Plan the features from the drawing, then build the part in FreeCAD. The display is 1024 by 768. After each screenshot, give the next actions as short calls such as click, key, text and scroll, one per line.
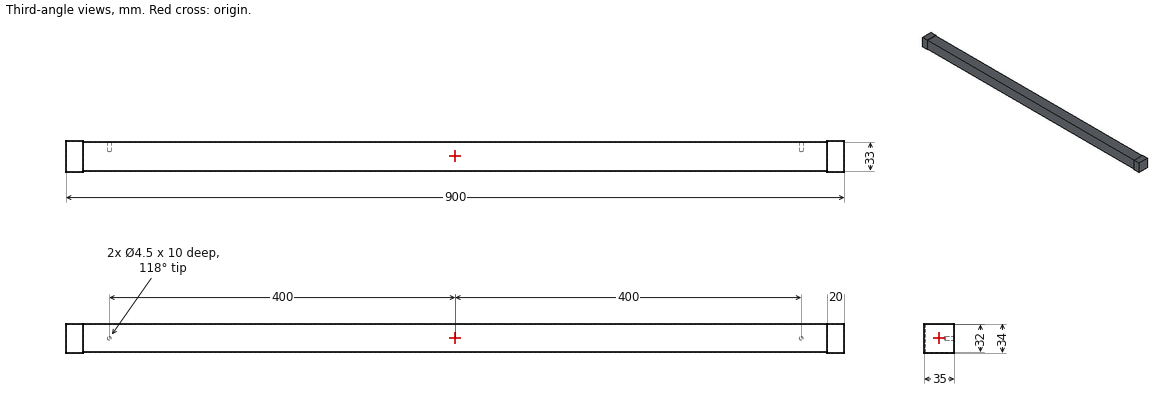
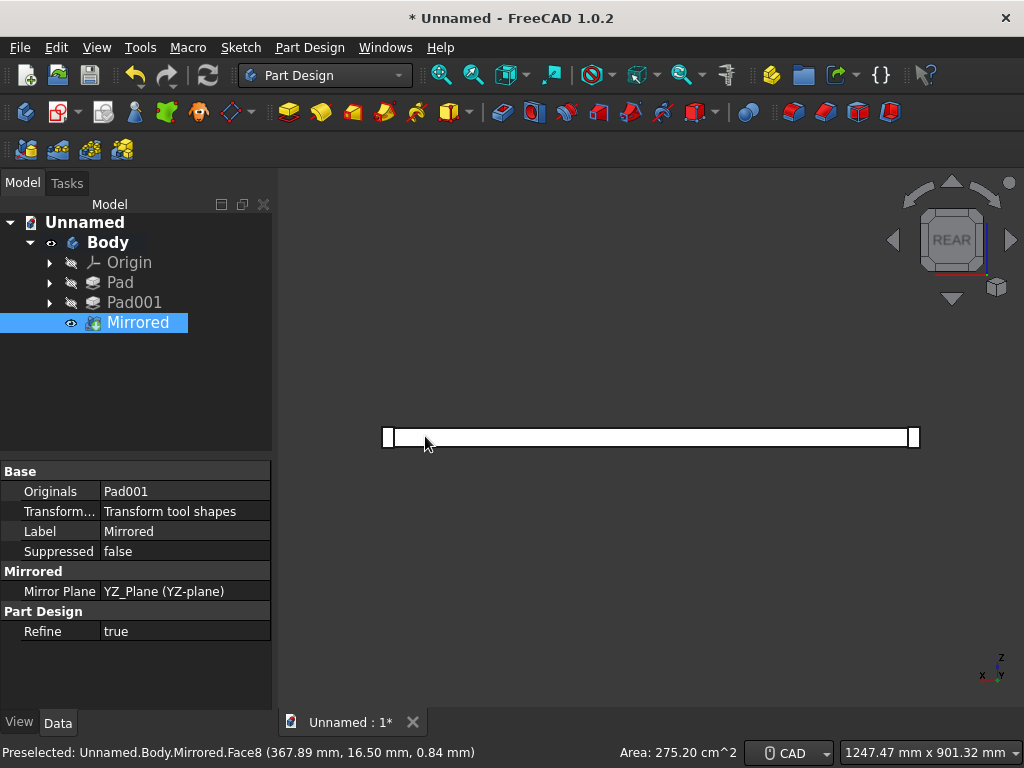
click(58, 112)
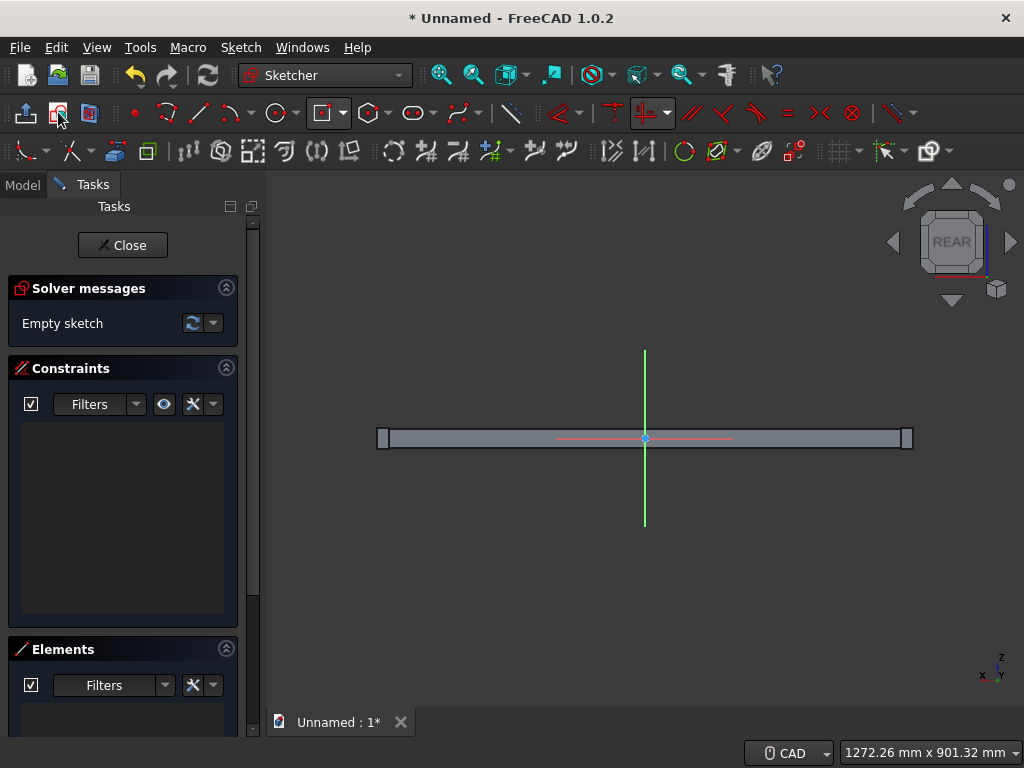
scroll(294, 439, down, 1)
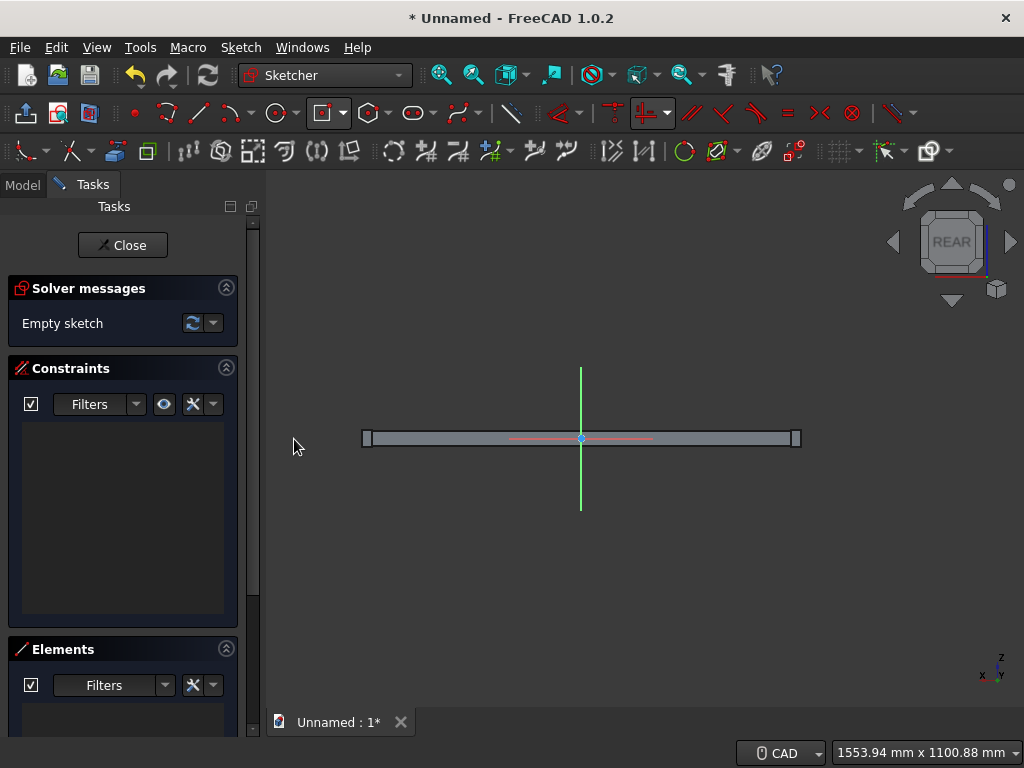
click(276, 114)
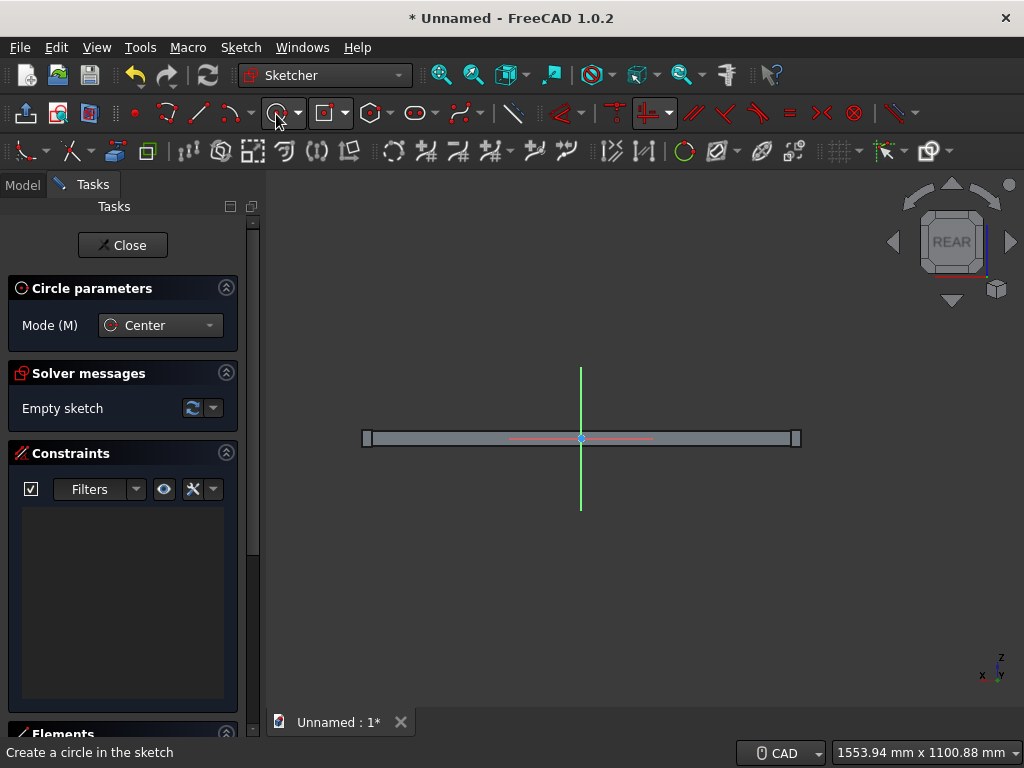
scroll(776, 439, up, 16)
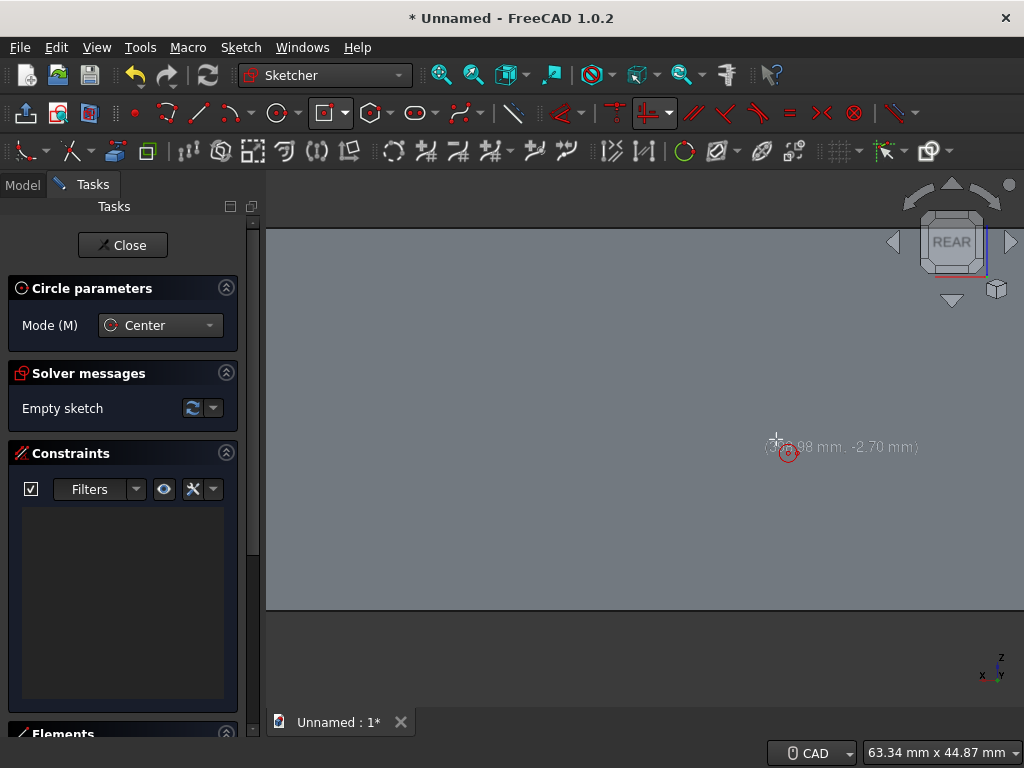
scroll(817, 440, down, 15)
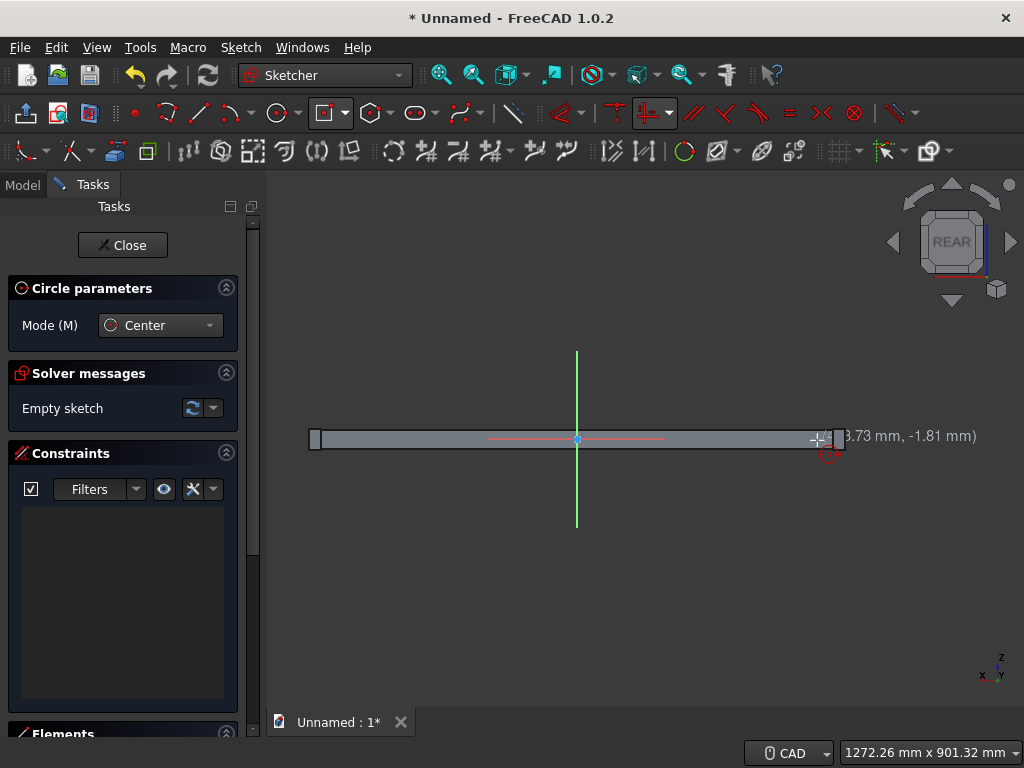
click(815, 439)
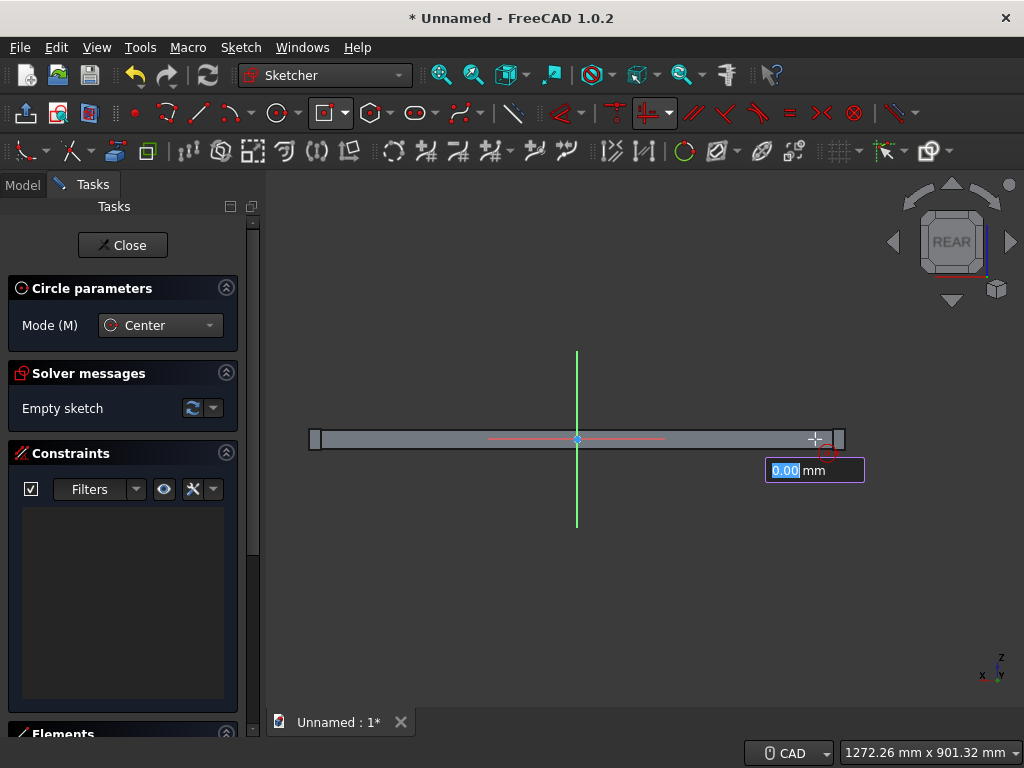
scroll(815, 441, up, 13)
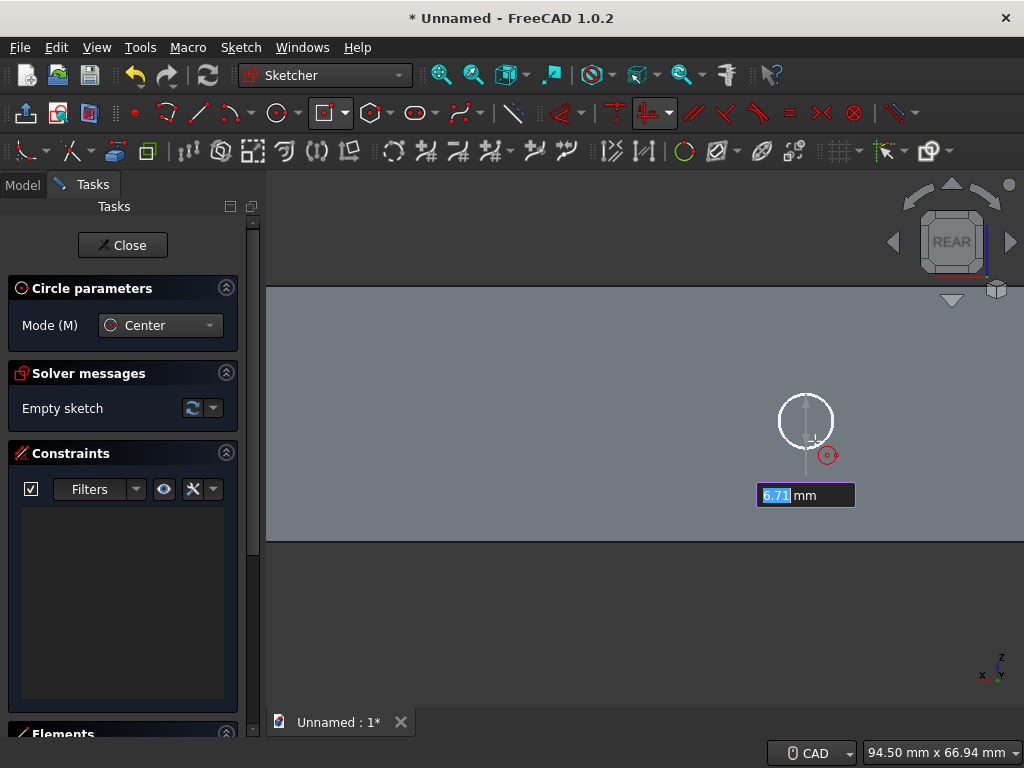
click(806, 431)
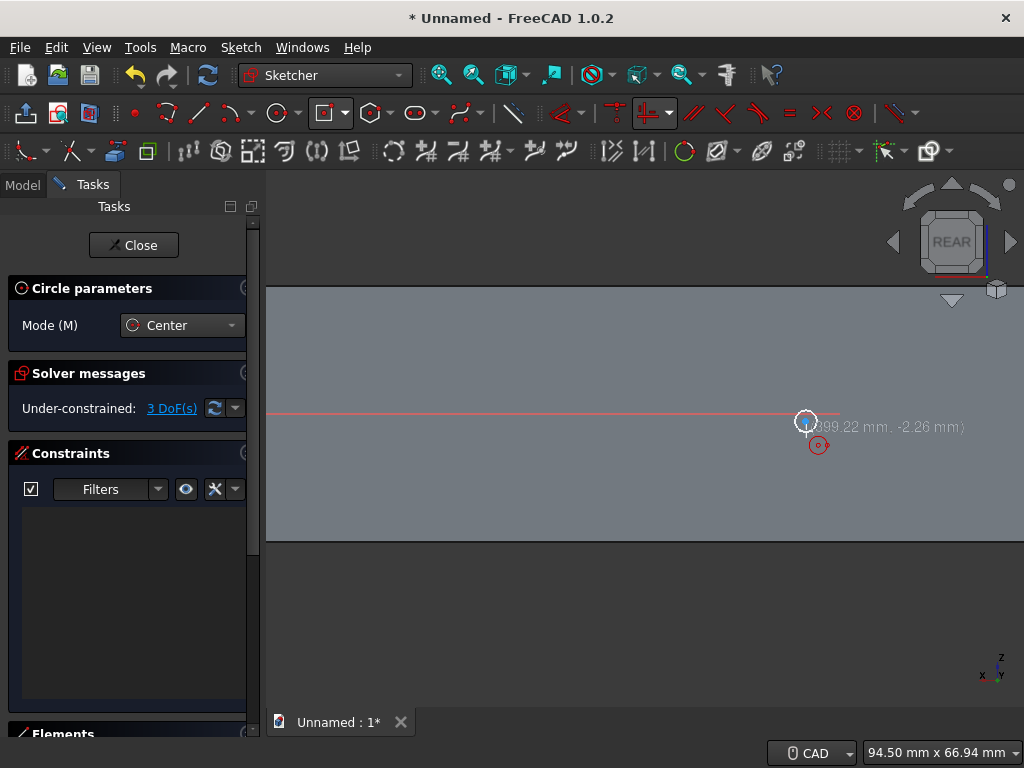
scroll(769, 440, down, 14)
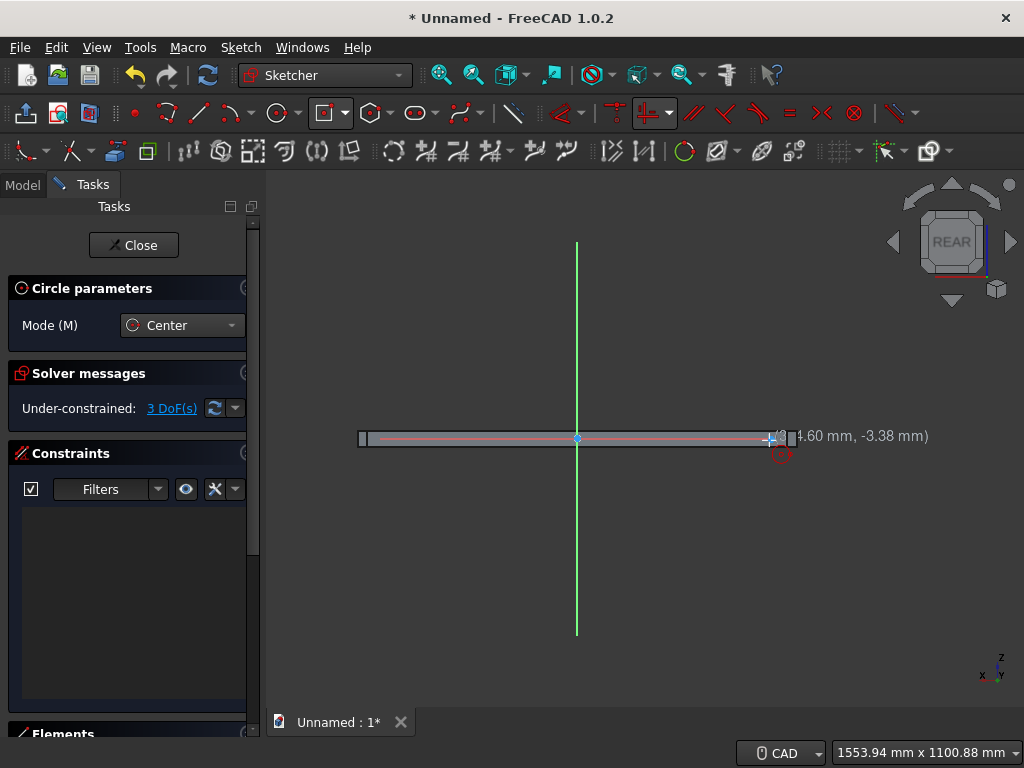
scroll(382, 439, up, 16)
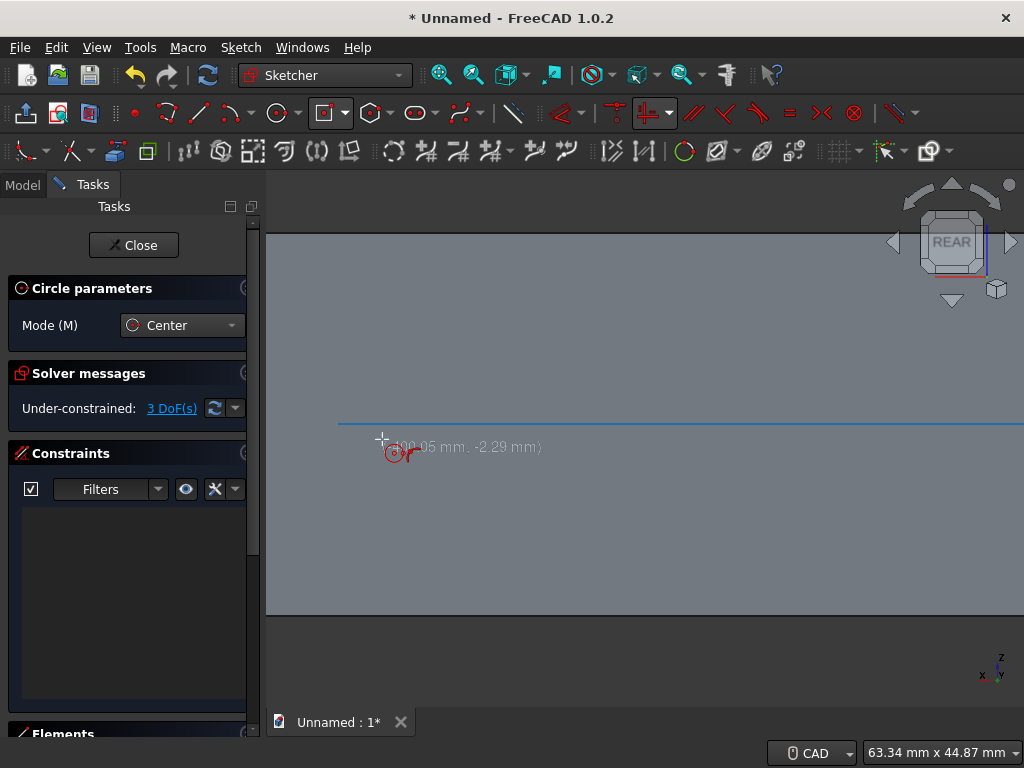
scroll(336, 439, down, 15)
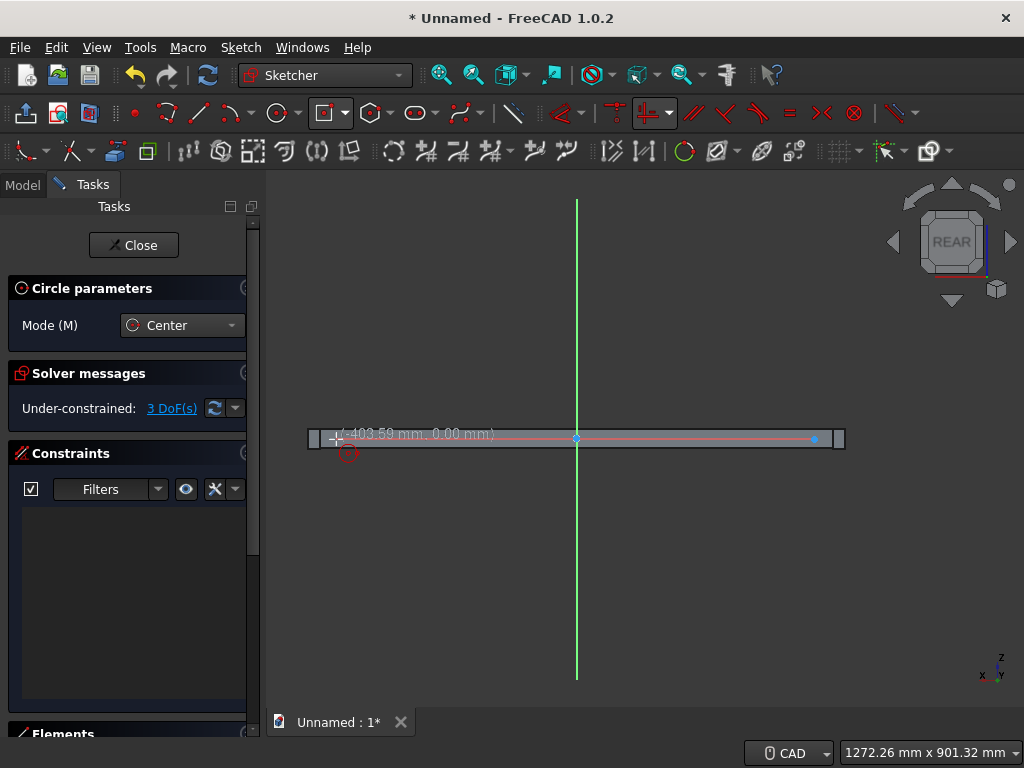
click(338, 439)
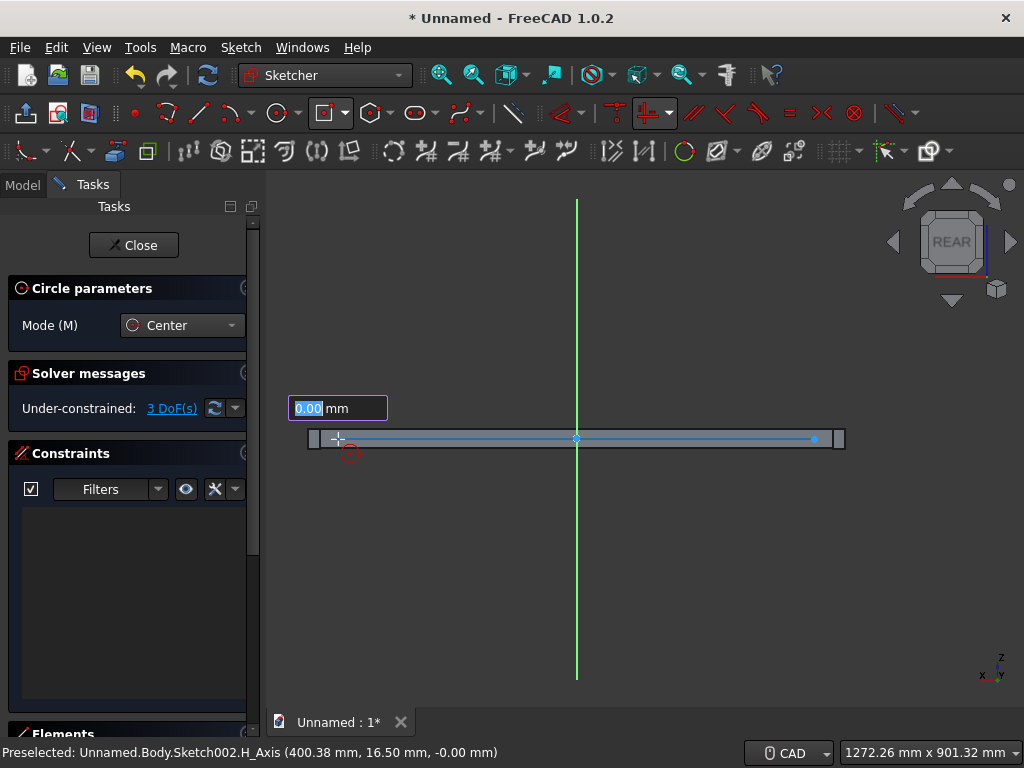
scroll(338, 440, up, 13)